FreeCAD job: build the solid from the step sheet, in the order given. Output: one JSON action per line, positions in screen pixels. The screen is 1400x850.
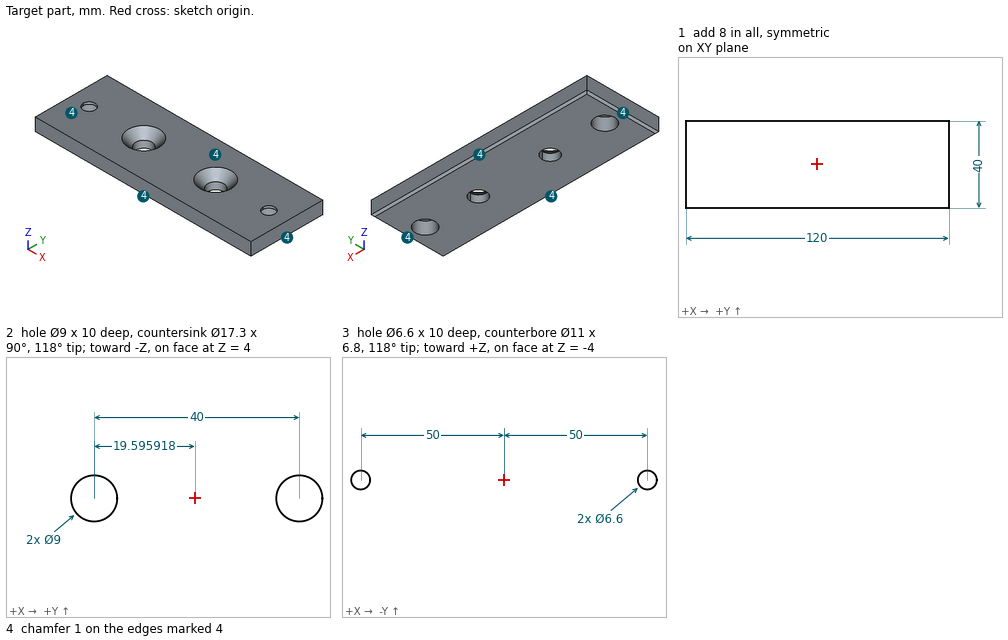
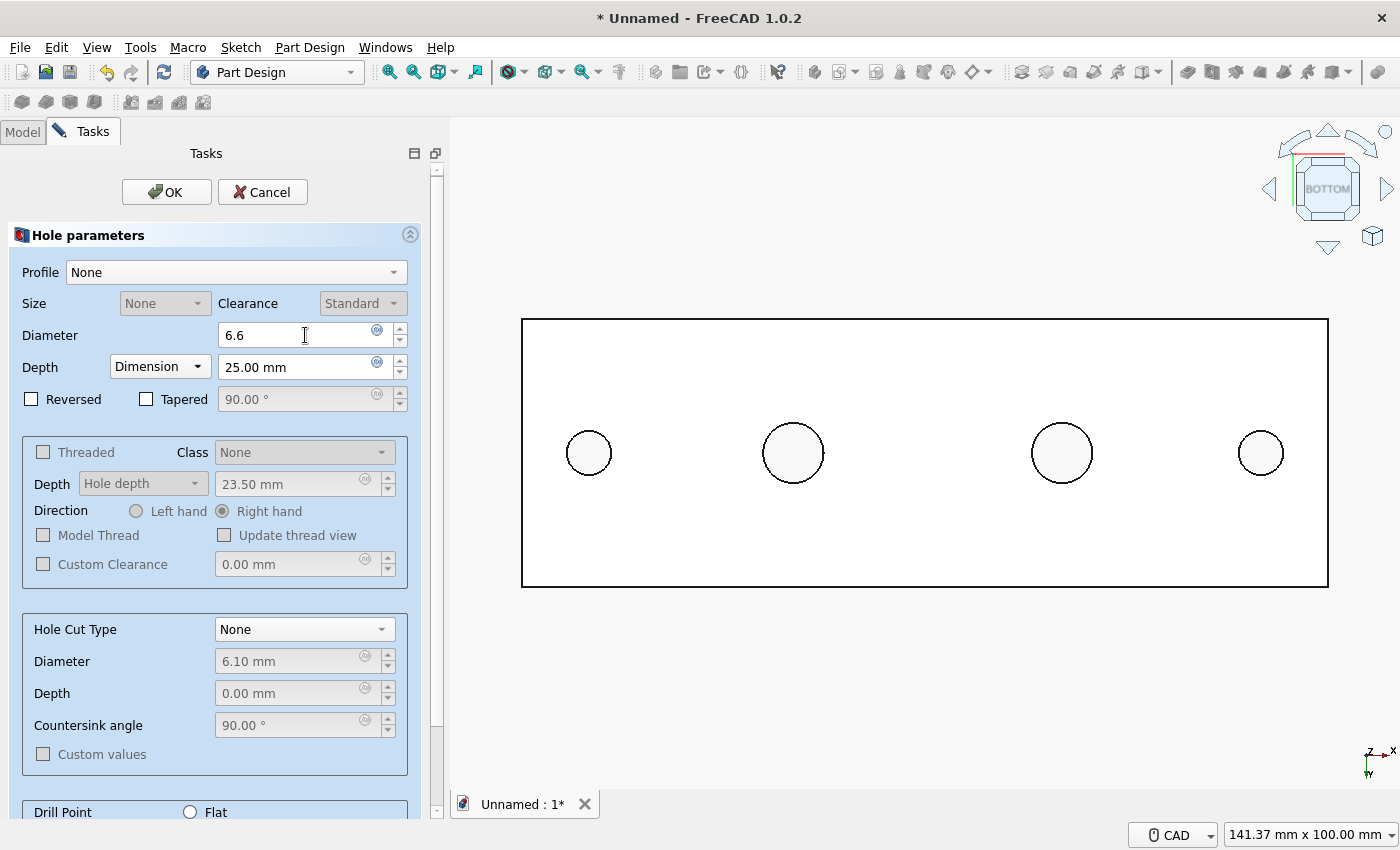
{"action": "triple_click", "coordinate": [305, 367]}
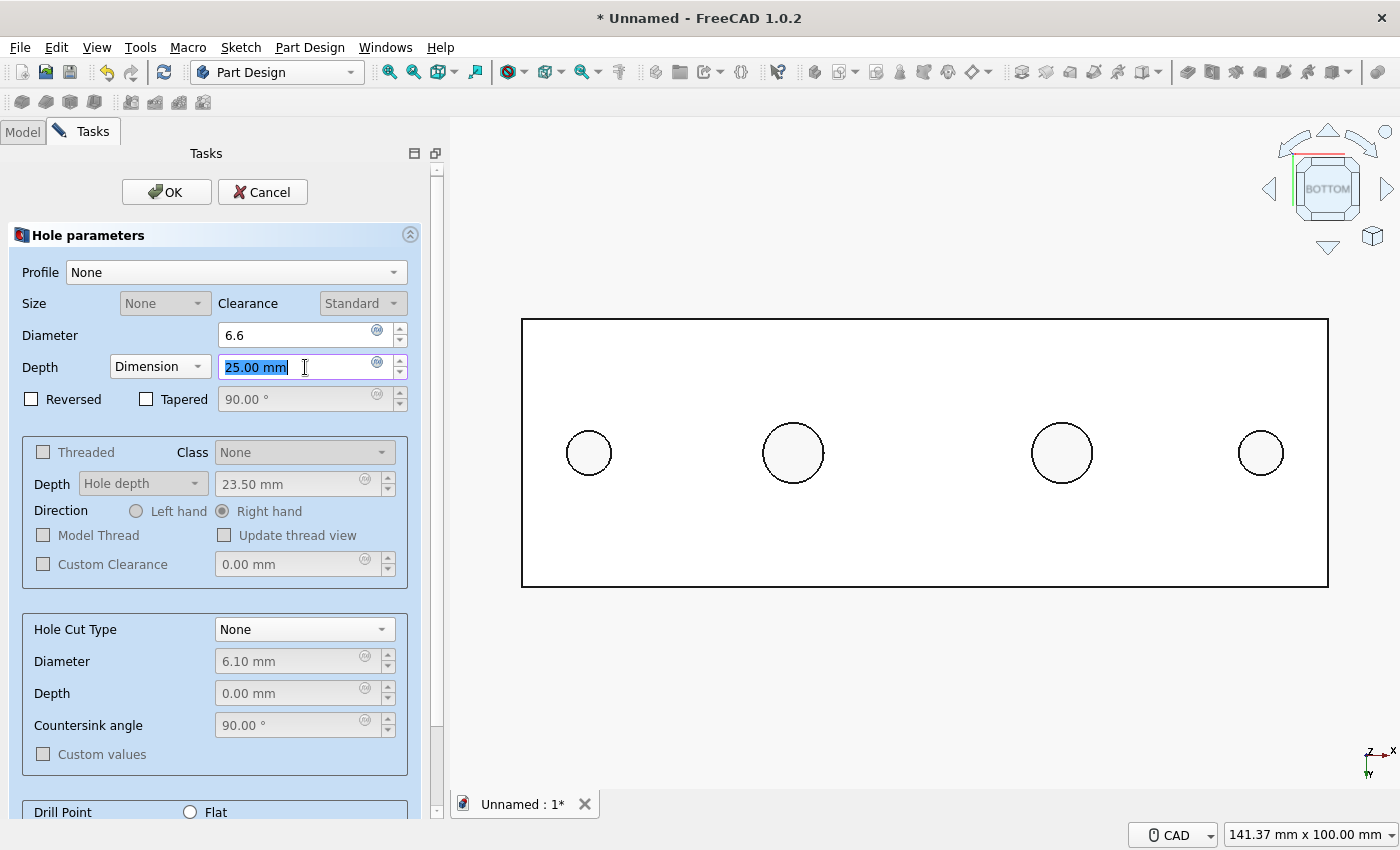
{"action": "type", "text": "10"}
{"action": "key", "text": "Tab"}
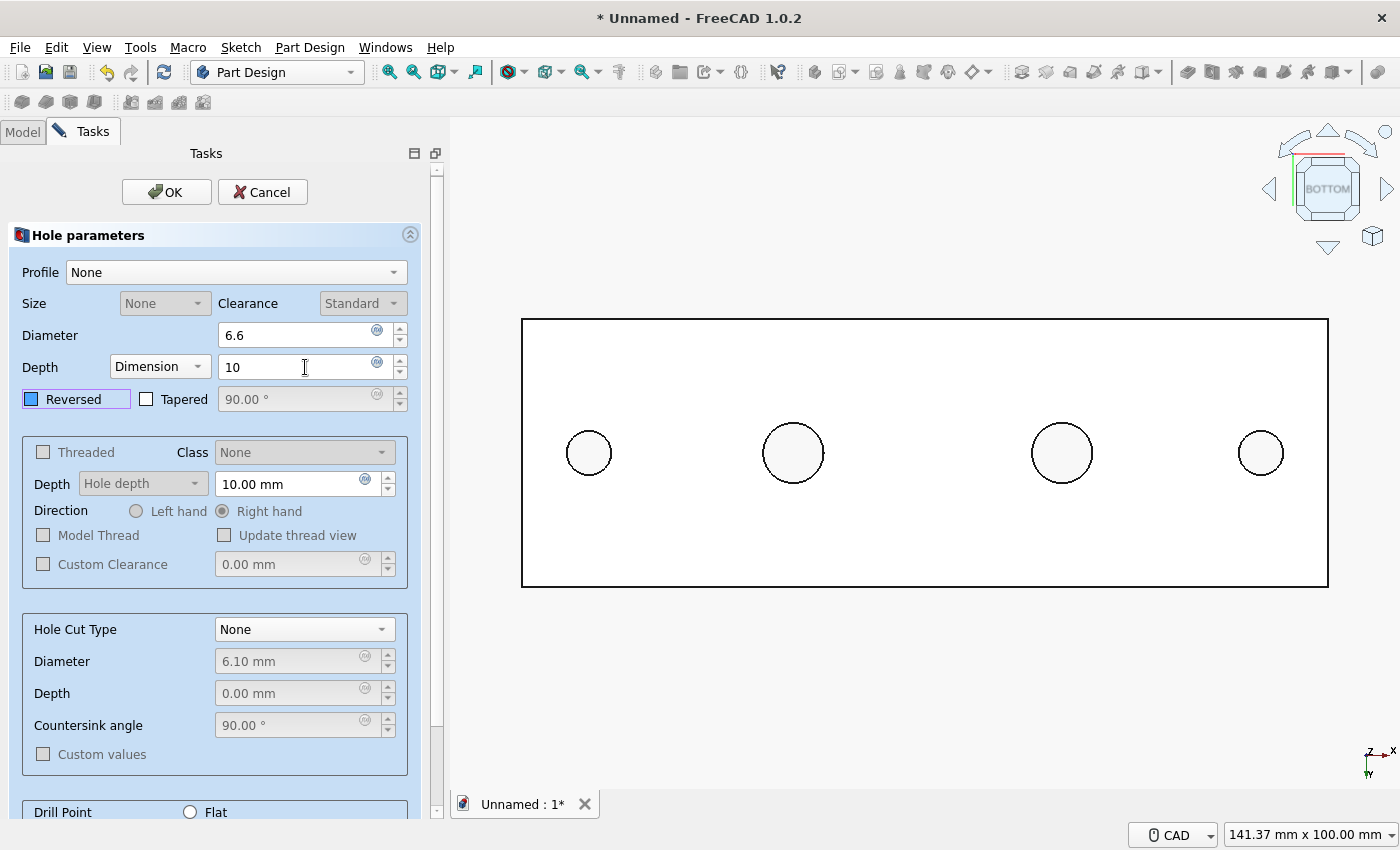
{"action": "left_click", "coordinate": [306, 630]}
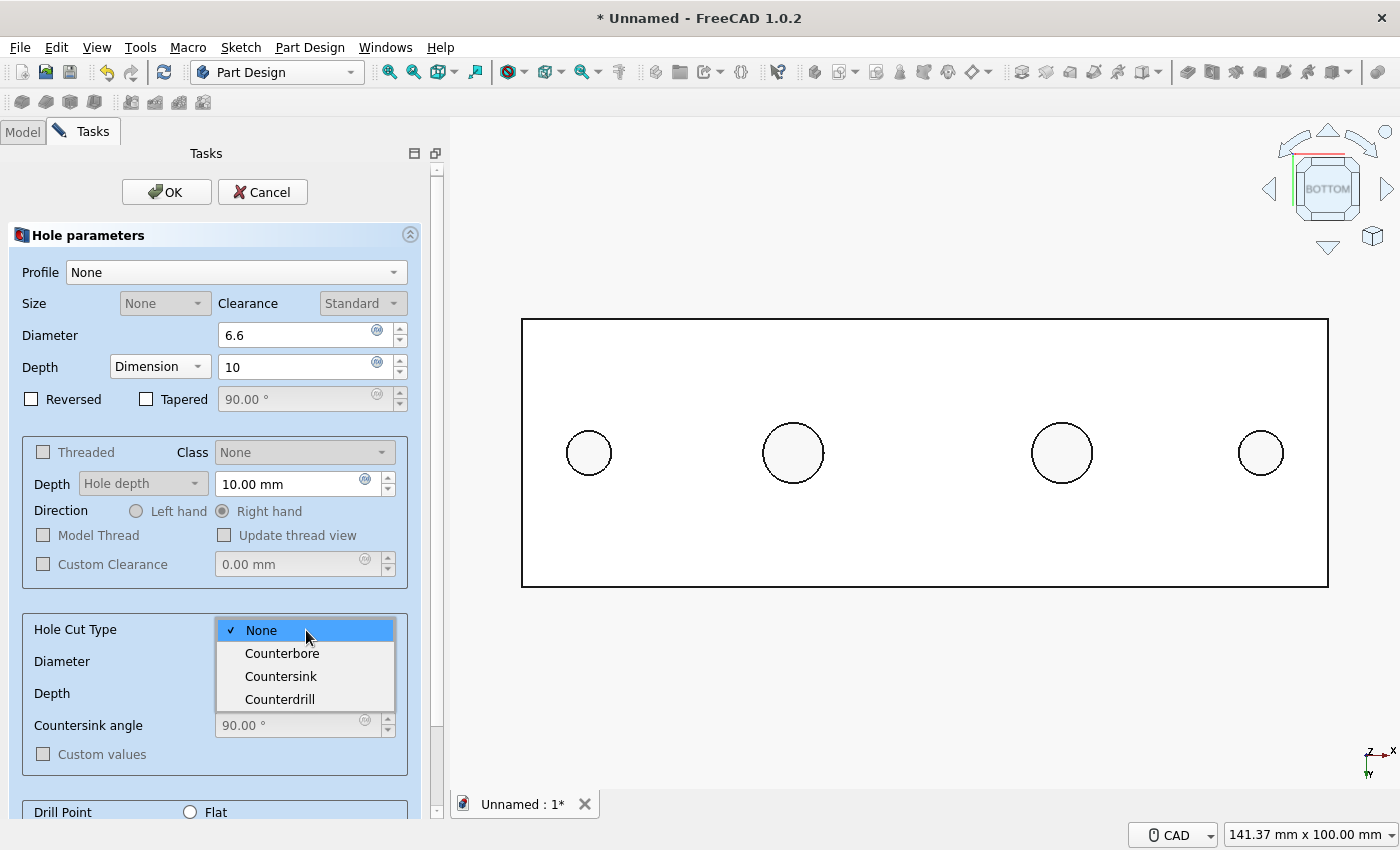
{"action": "left_click", "coordinate": [304, 654]}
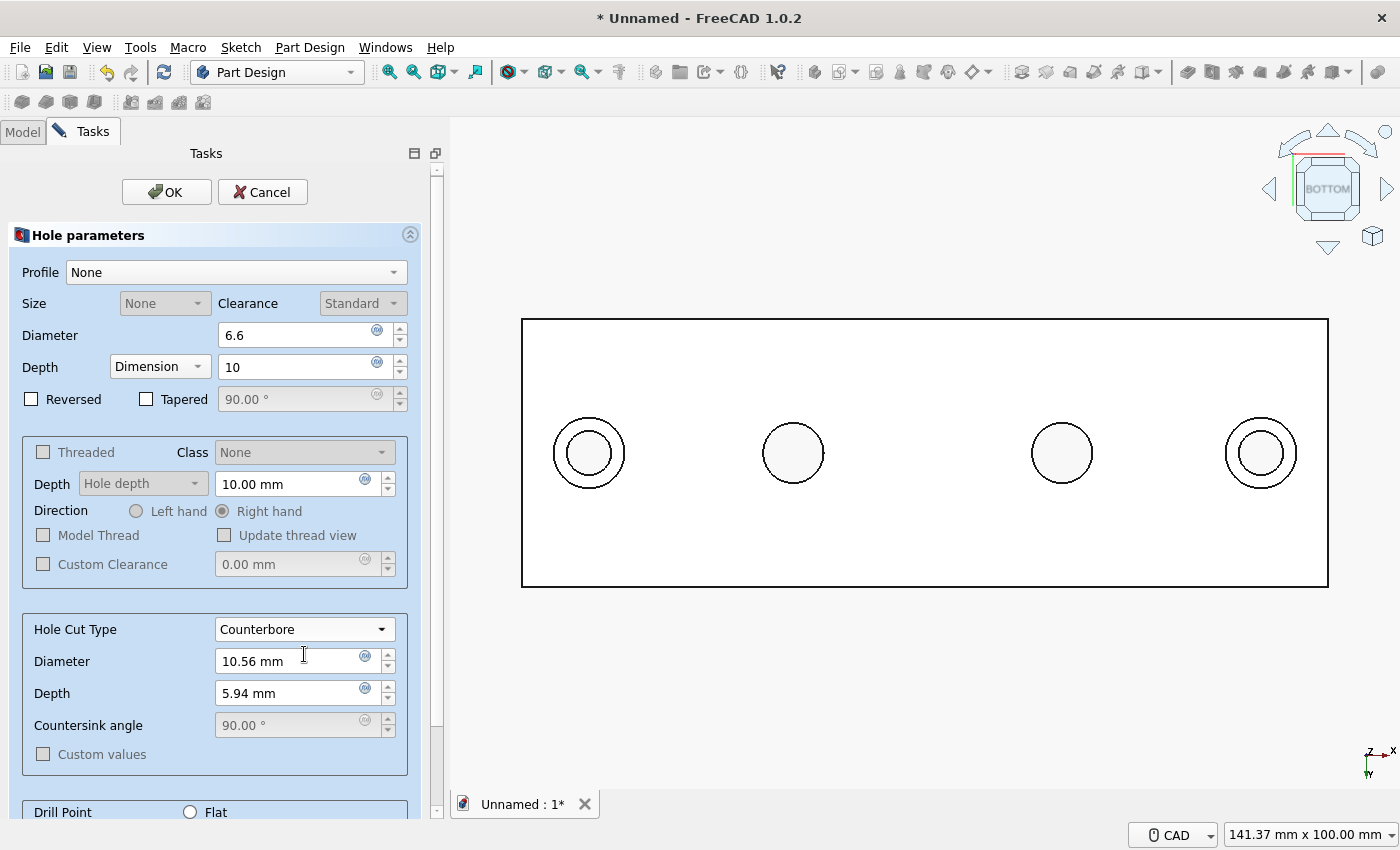
{"action": "triple_click", "coordinate": [298, 661]}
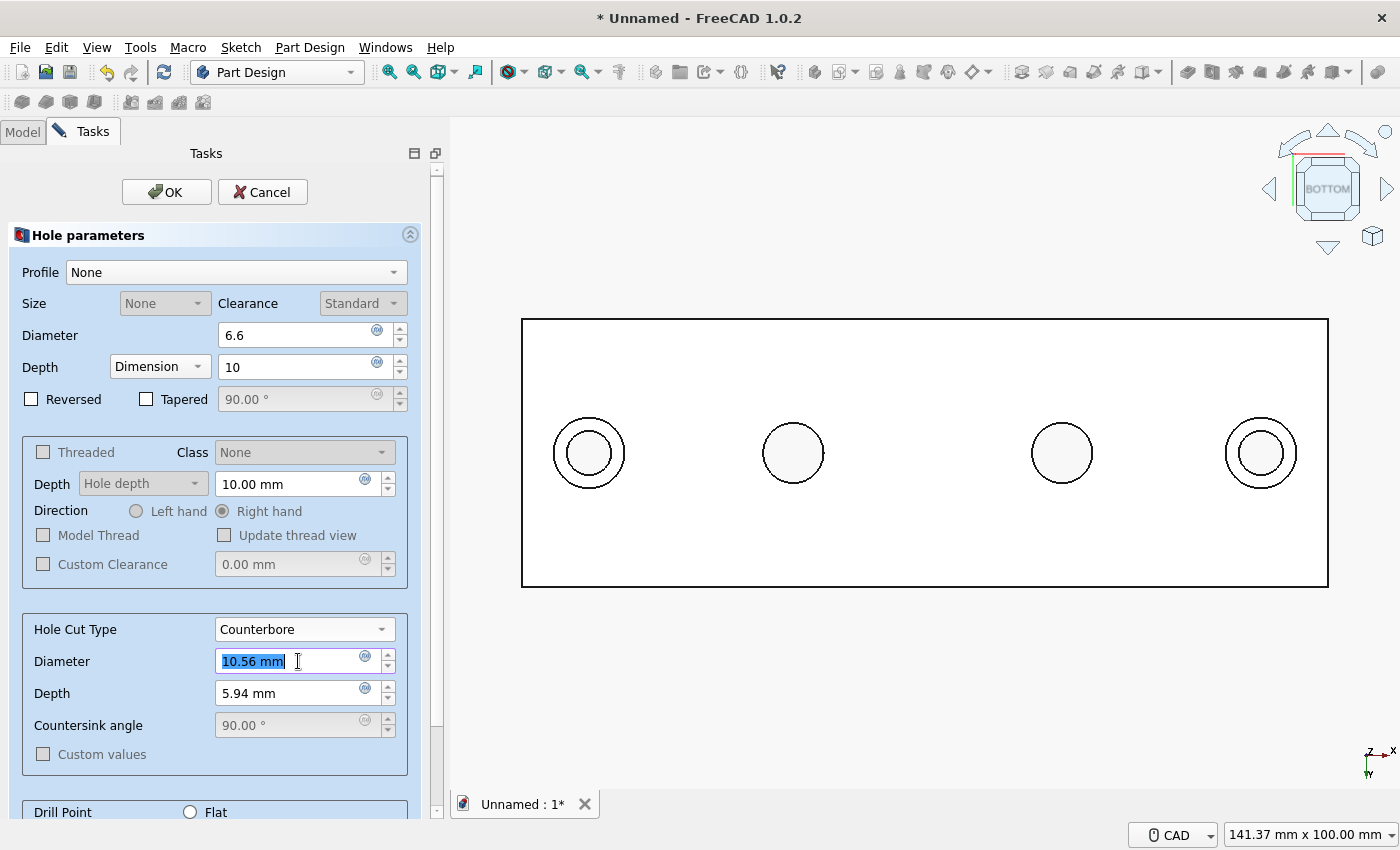
{"action": "type", "text": "11"}
{"action": "key", "text": "Tab"}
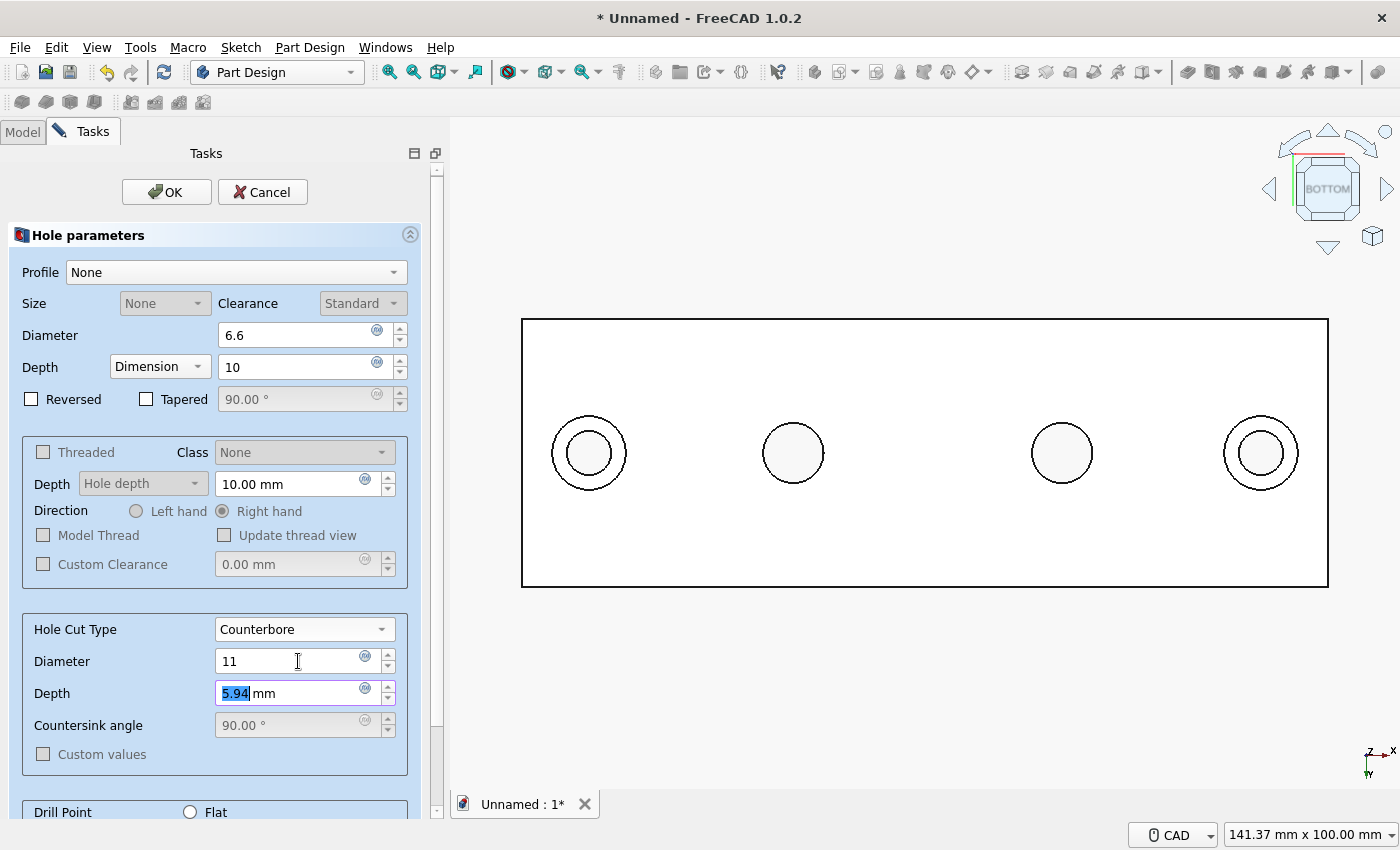
{"action": "type", "text": "6.8"}
{"action": "key", "text": "Tab"}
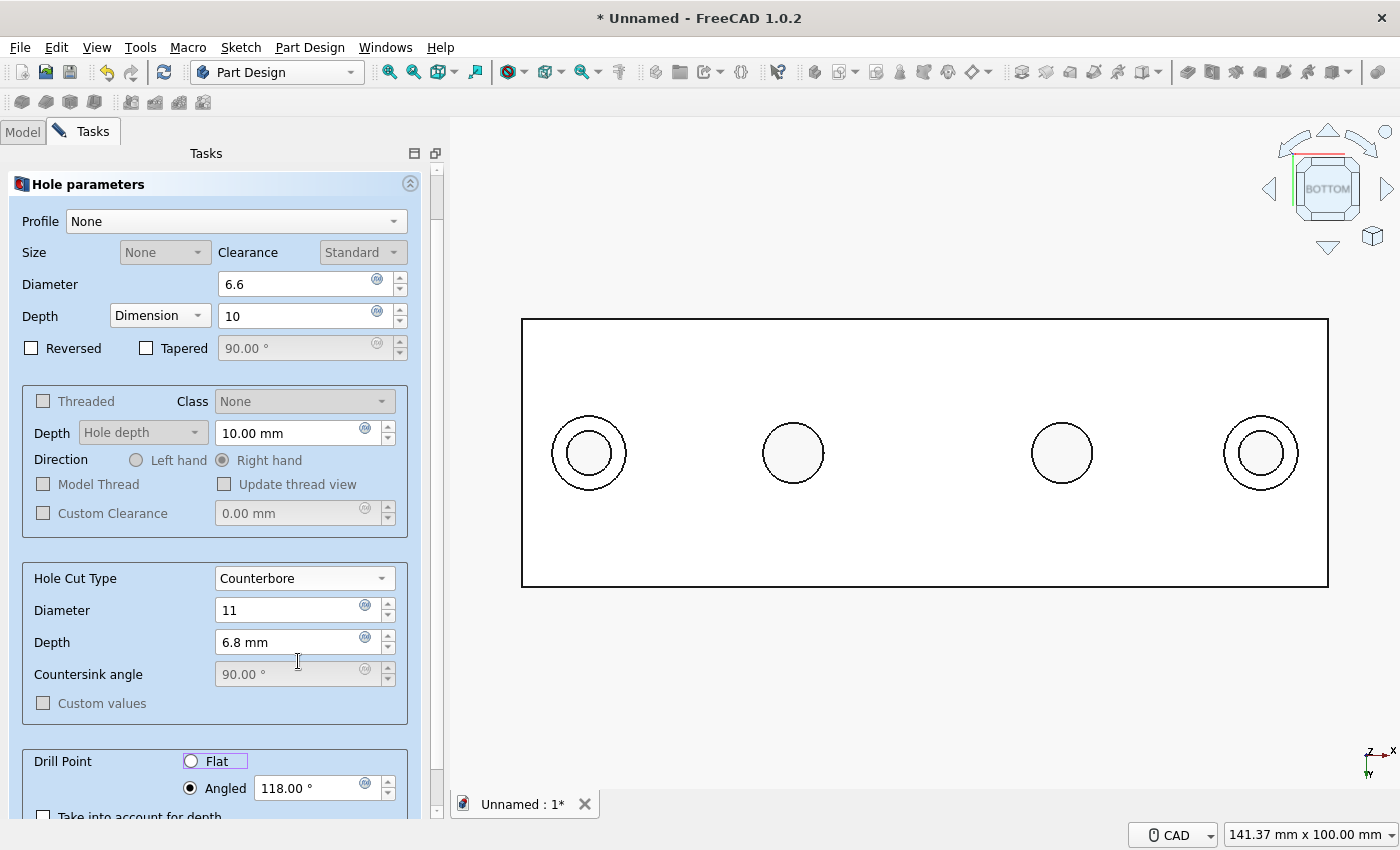
{"action": "scroll", "coordinate": [437, 490], "scroll_direction": "up", "scroll_amount": 2}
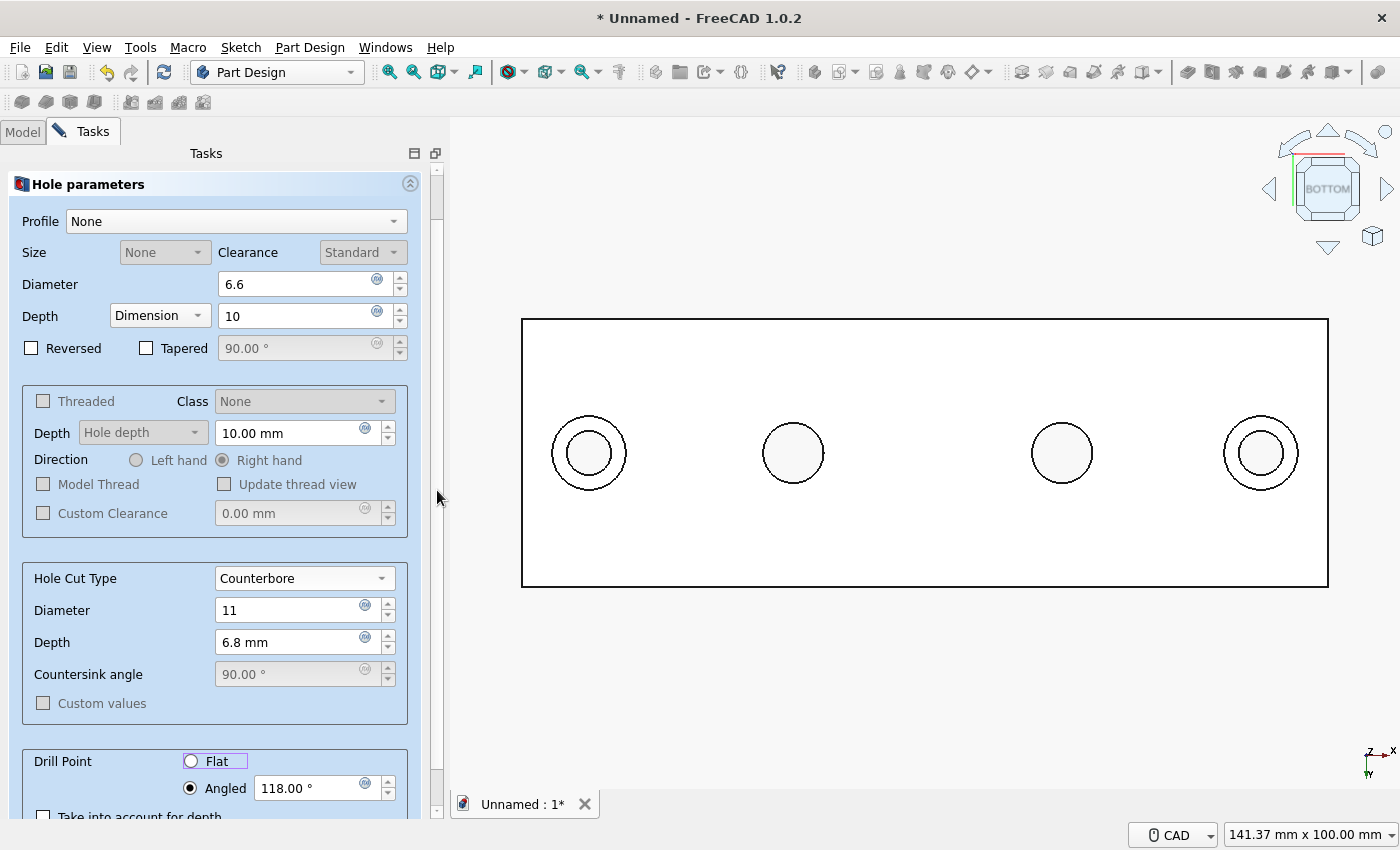
{"action": "left_click", "coordinate": [167, 192]}